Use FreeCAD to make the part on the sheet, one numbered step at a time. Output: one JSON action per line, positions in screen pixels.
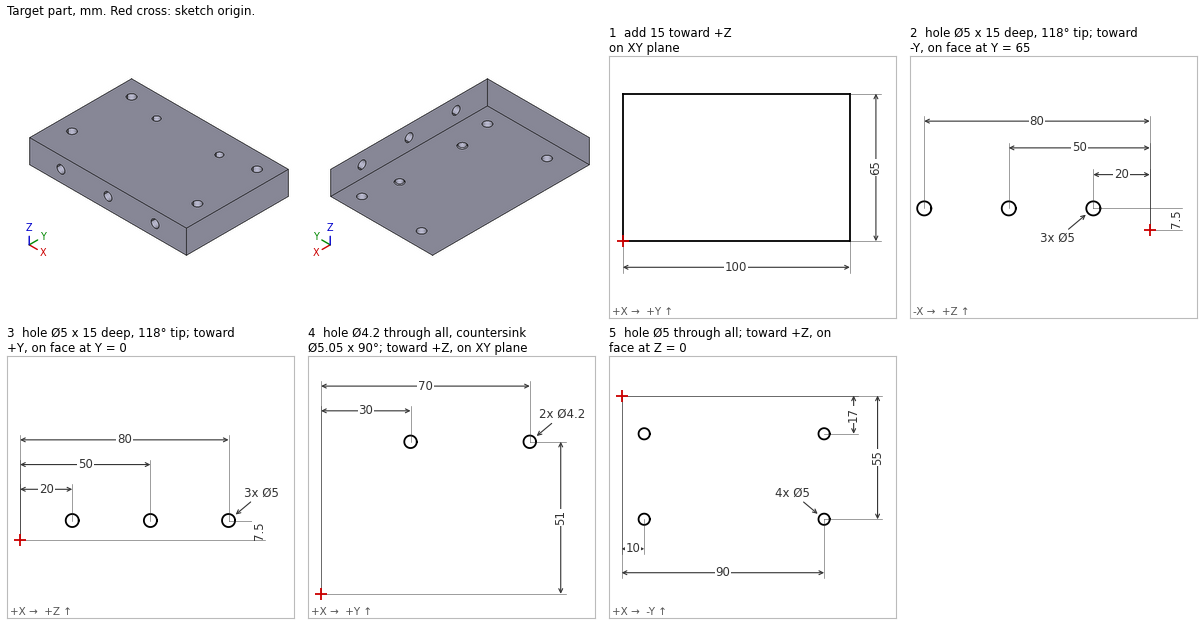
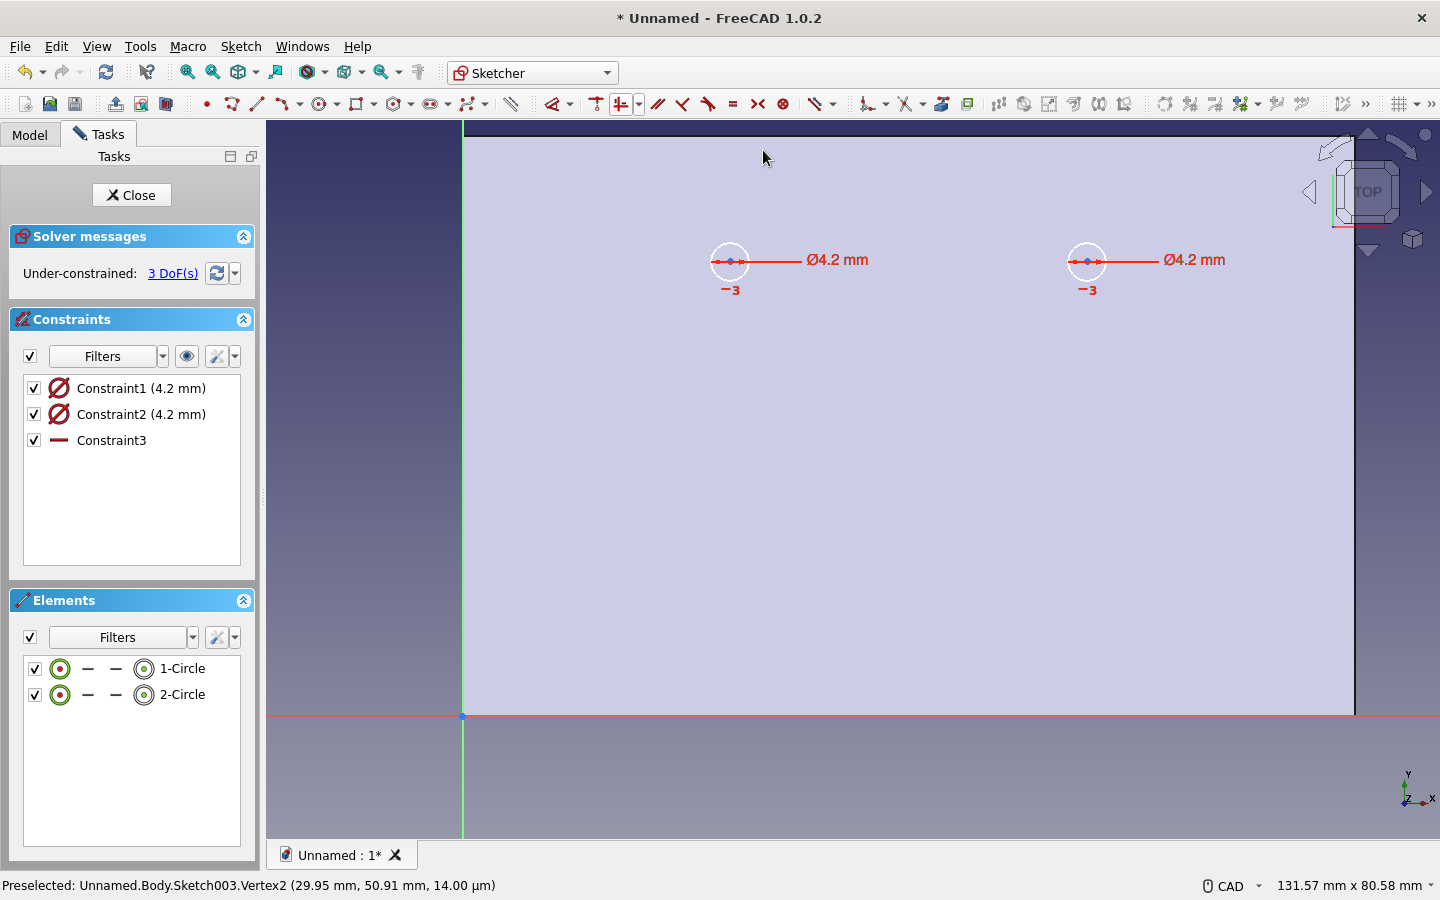
{"action": "left_click", "coordinate": [552, 104]}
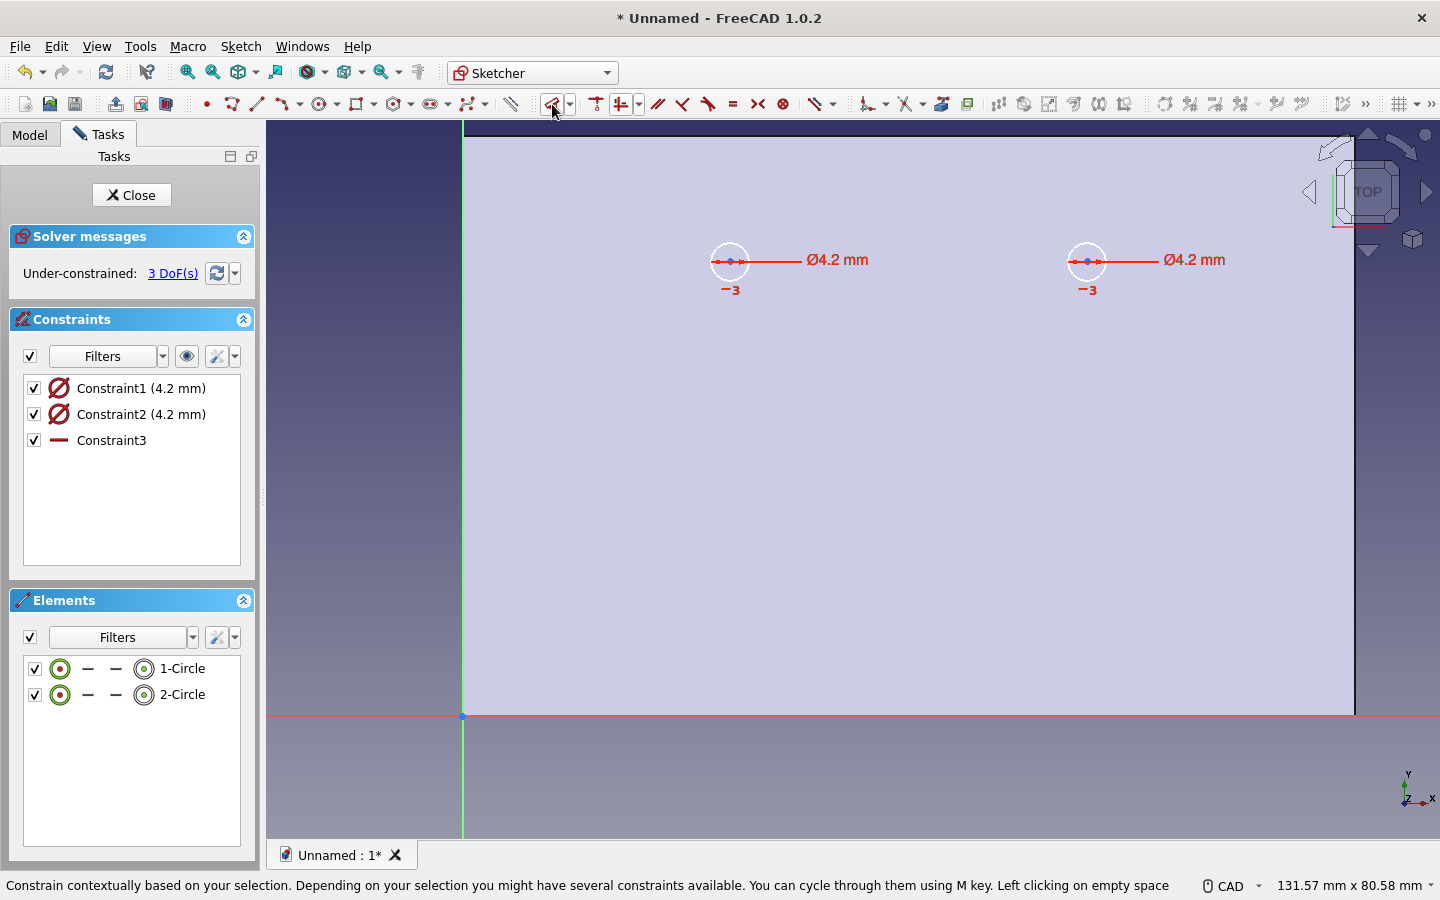
{"action": "left_click", "coordinate": [1087, 262]}
{"action": "left_click", "coordinate": [775, 750]}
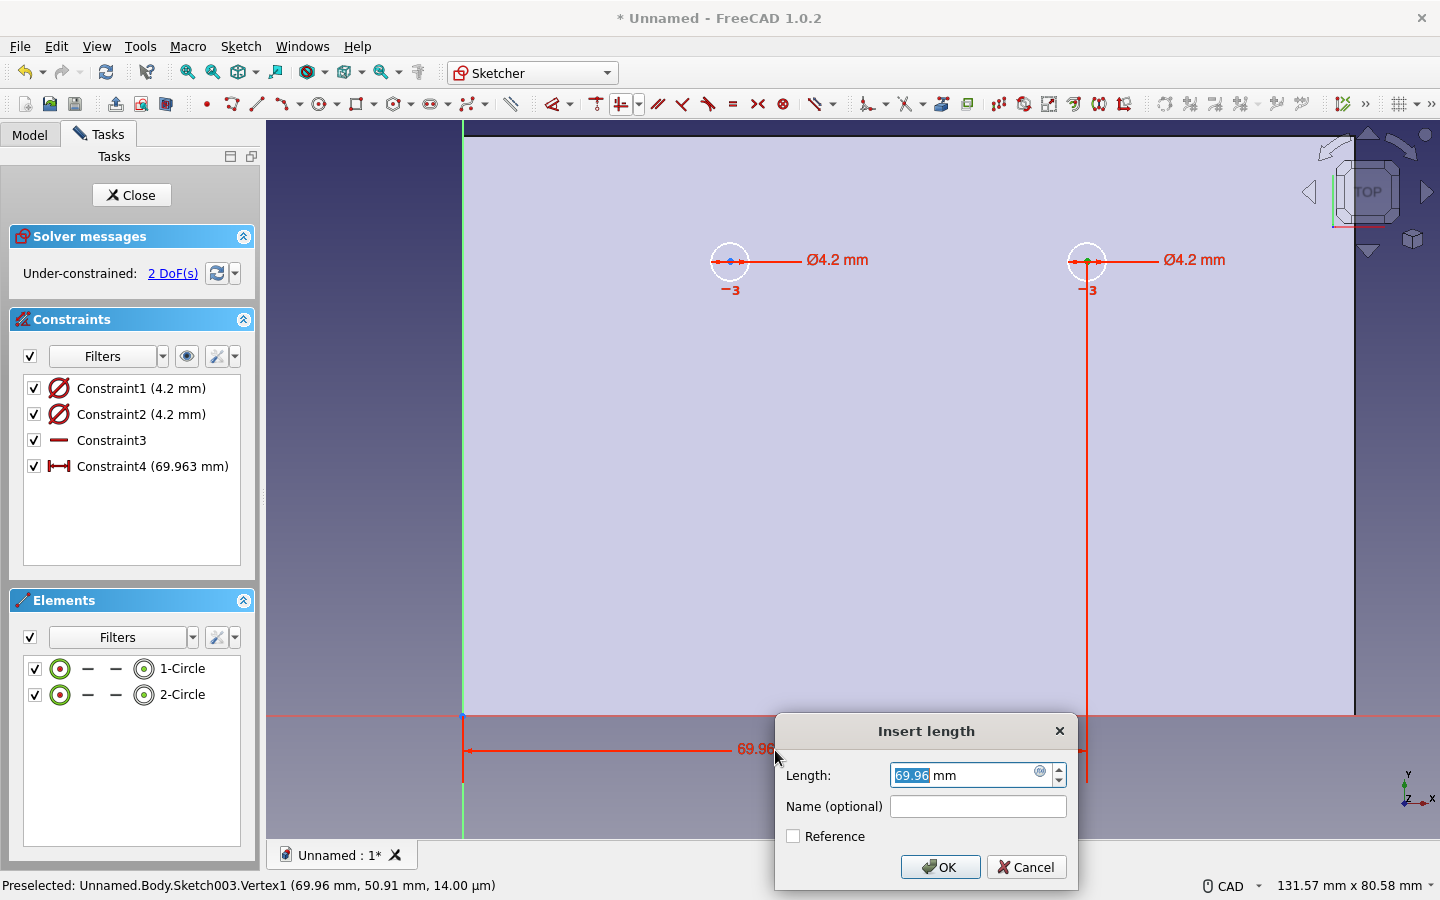
{"action": "type", "text": "70"}
{"action": "key", "text": "Return"}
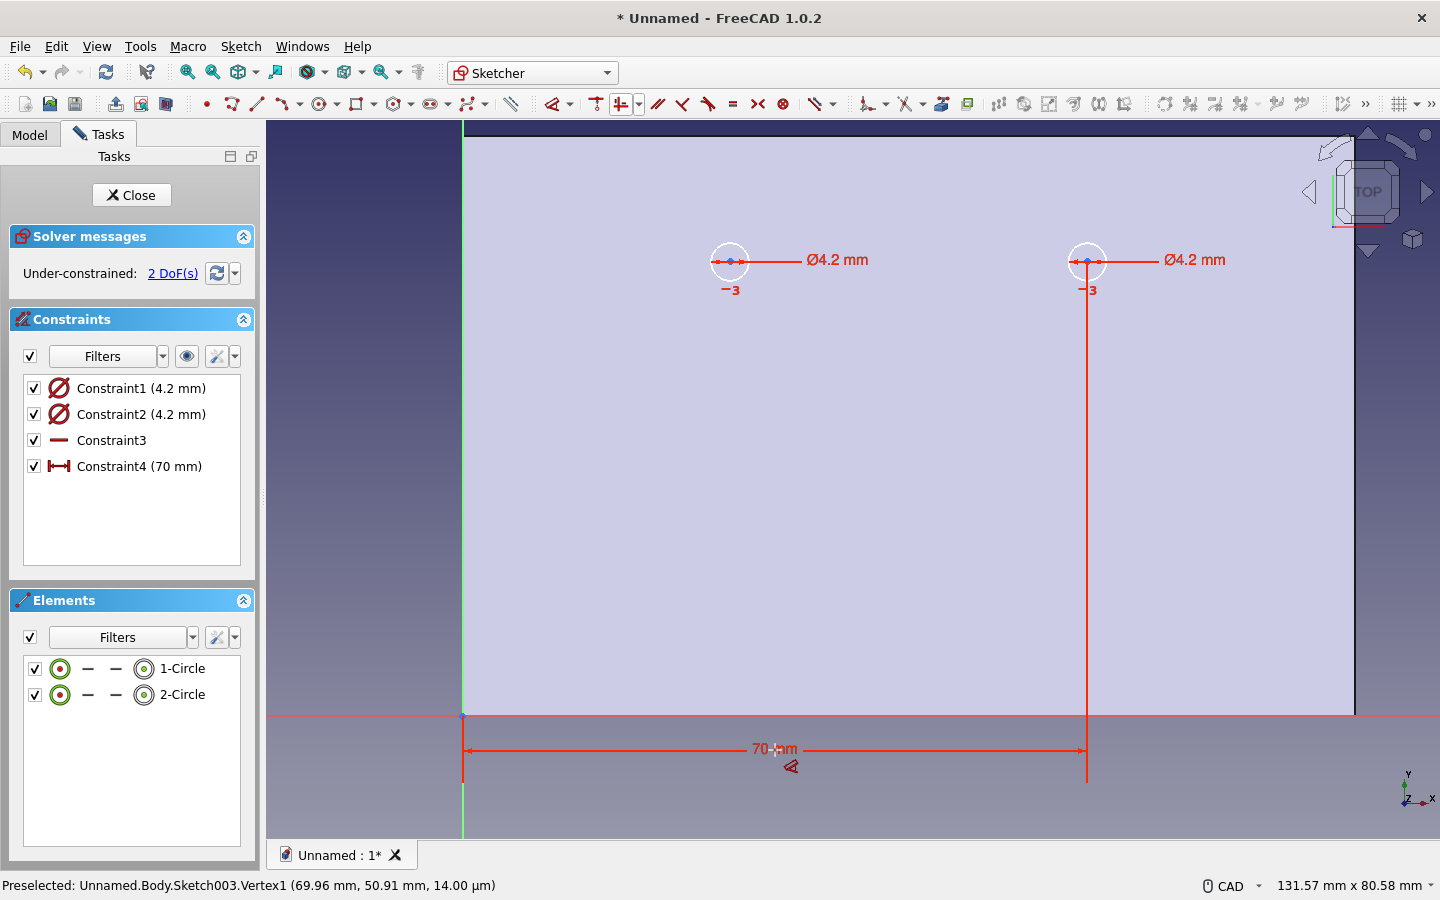
{"action": "left_click", "coordinate": [1087, 262]}
{"action": "left_click", "coordinate": [429, 489]}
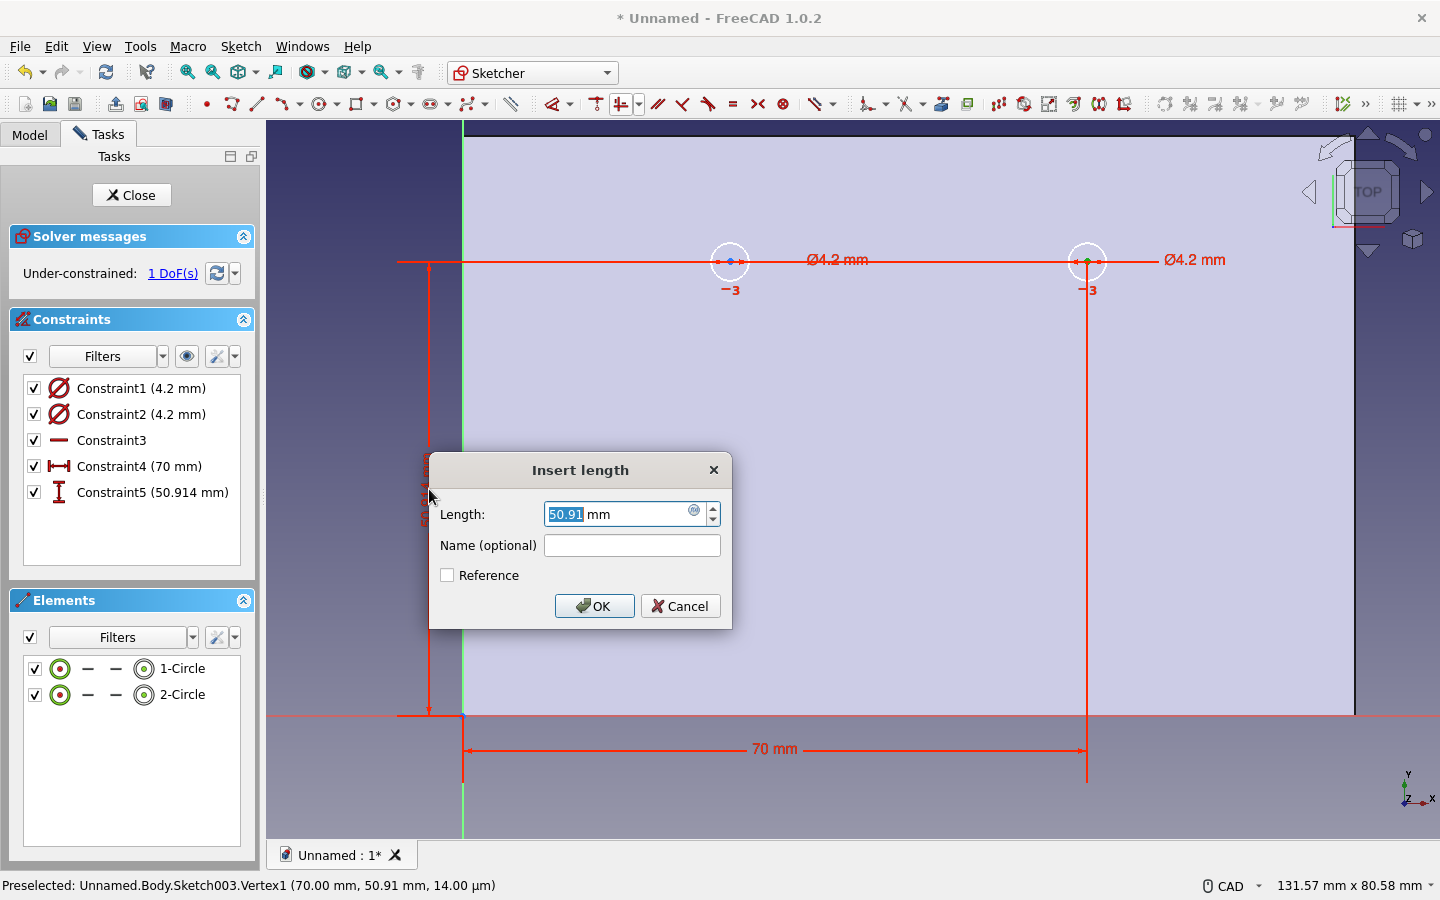
{"action": "type", "text": "51"}
{"action": "key", "text": "Return"}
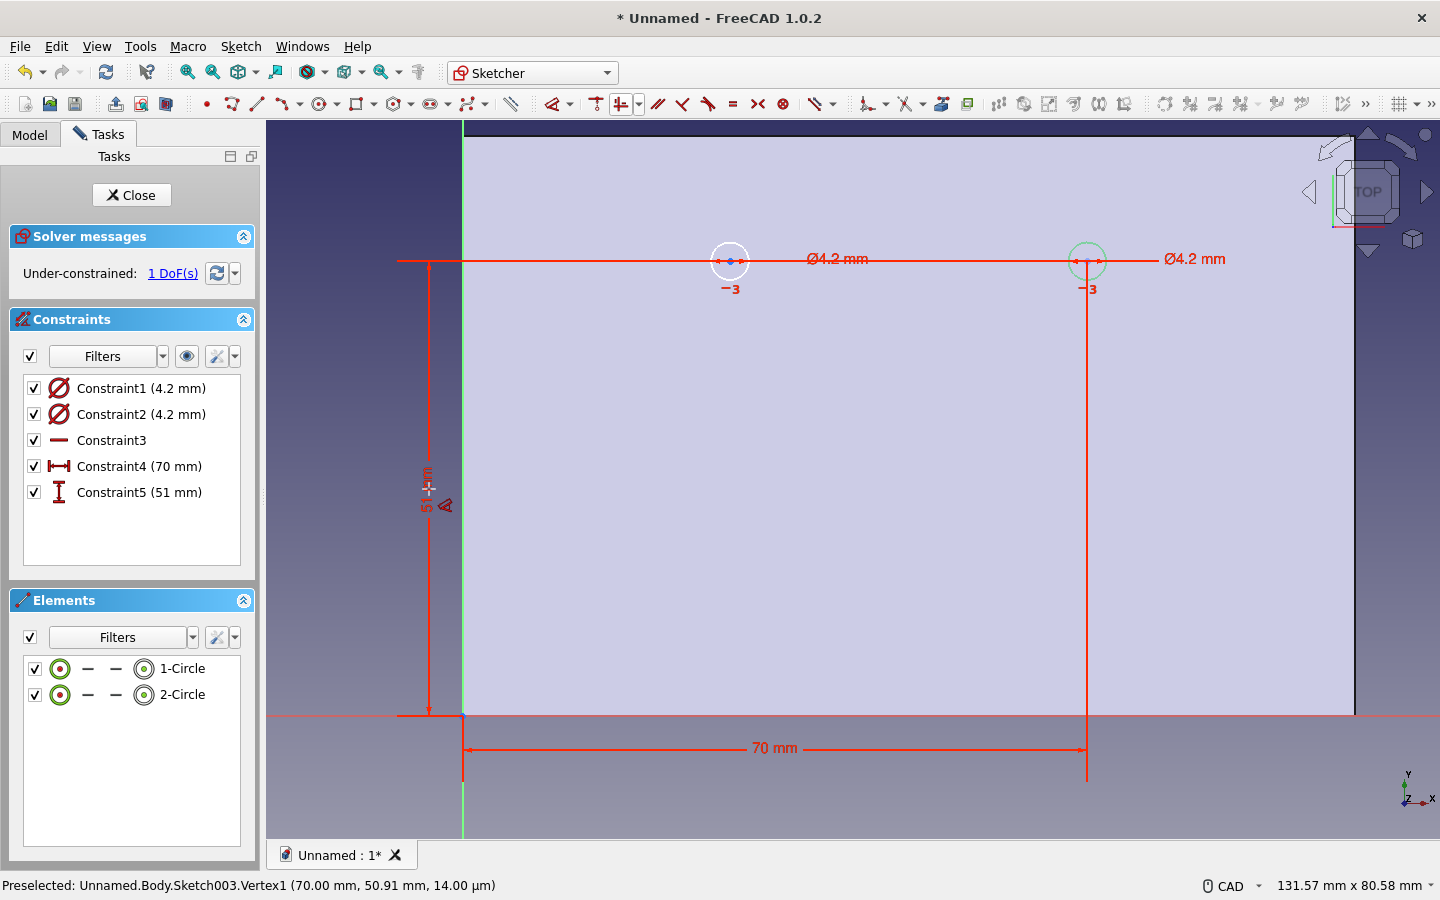
{"action": "left_click", "coordinate": [730, 261]}
{"action": "left_click", "coordinate": [596, 750]}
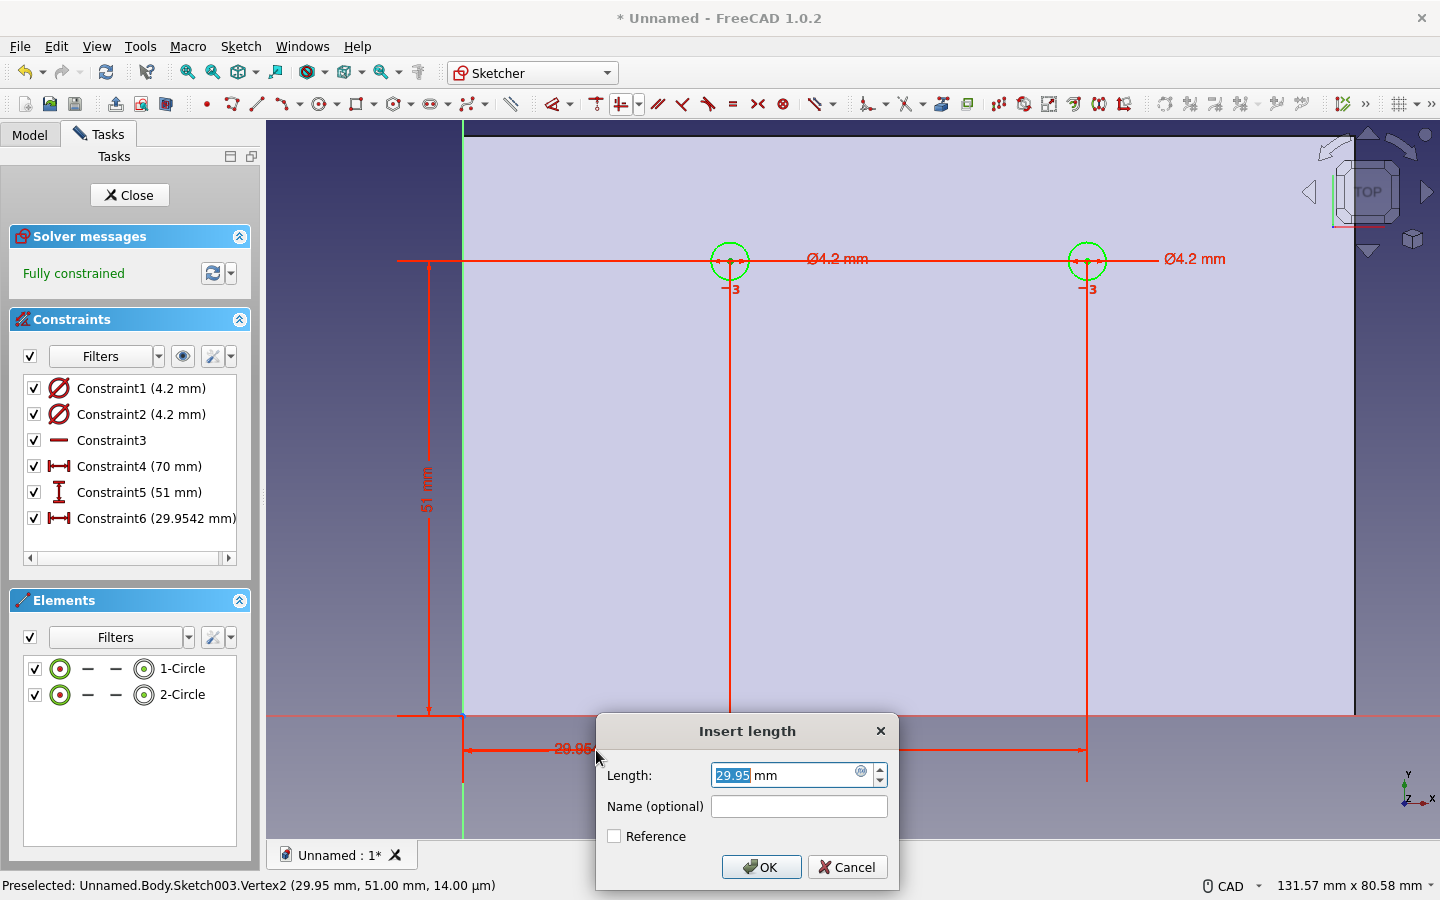
{"action": "type", "text": "30"}
{"action": "key", "text": "Return"}
{"action": "key", "text": "Escape"}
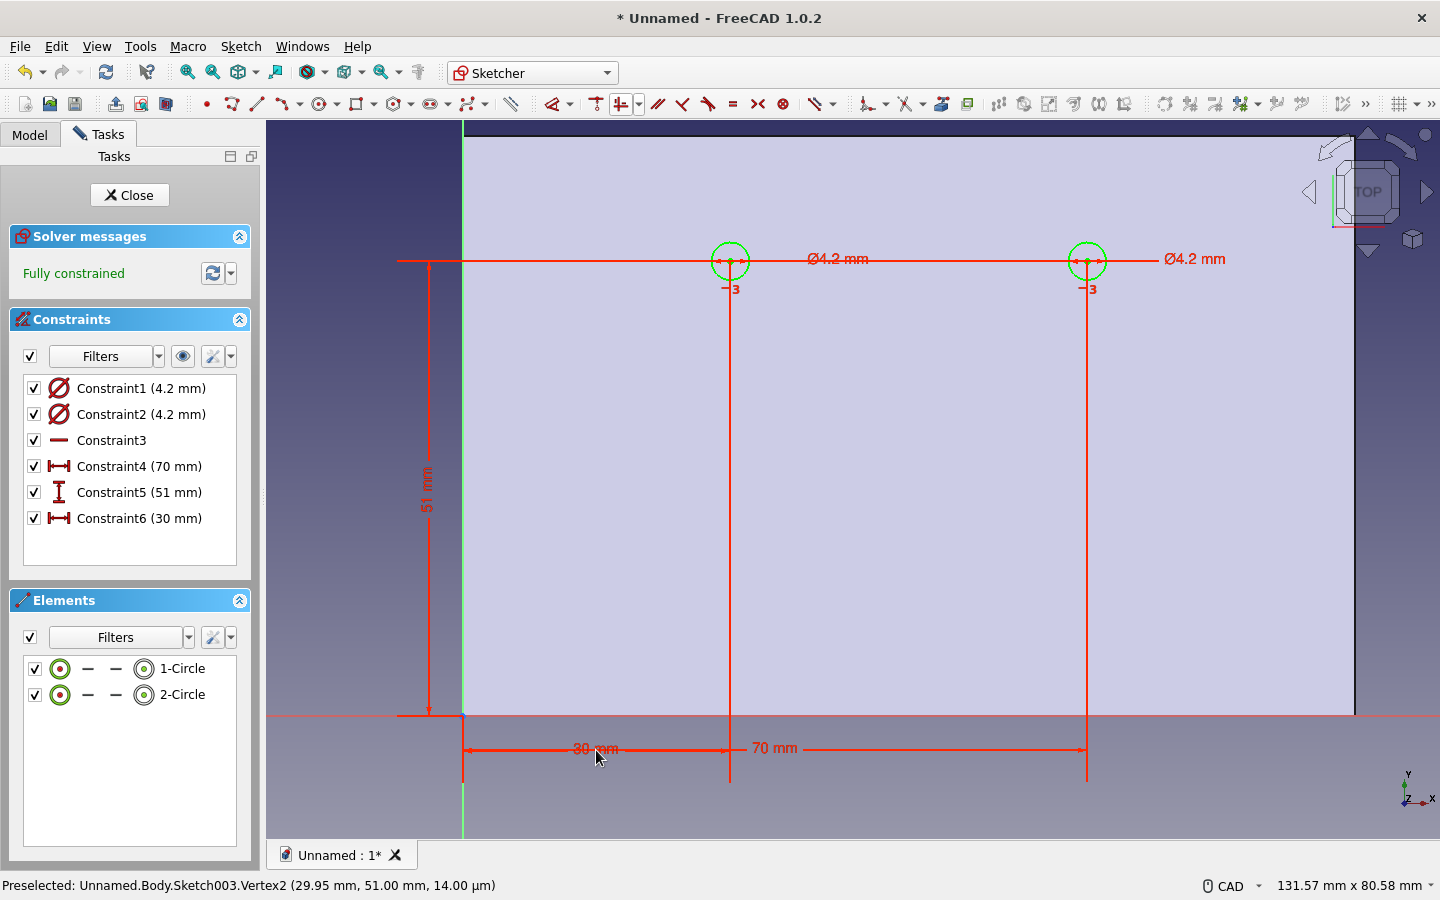
{"action": "left_click", "coordinate": [130, 195]}